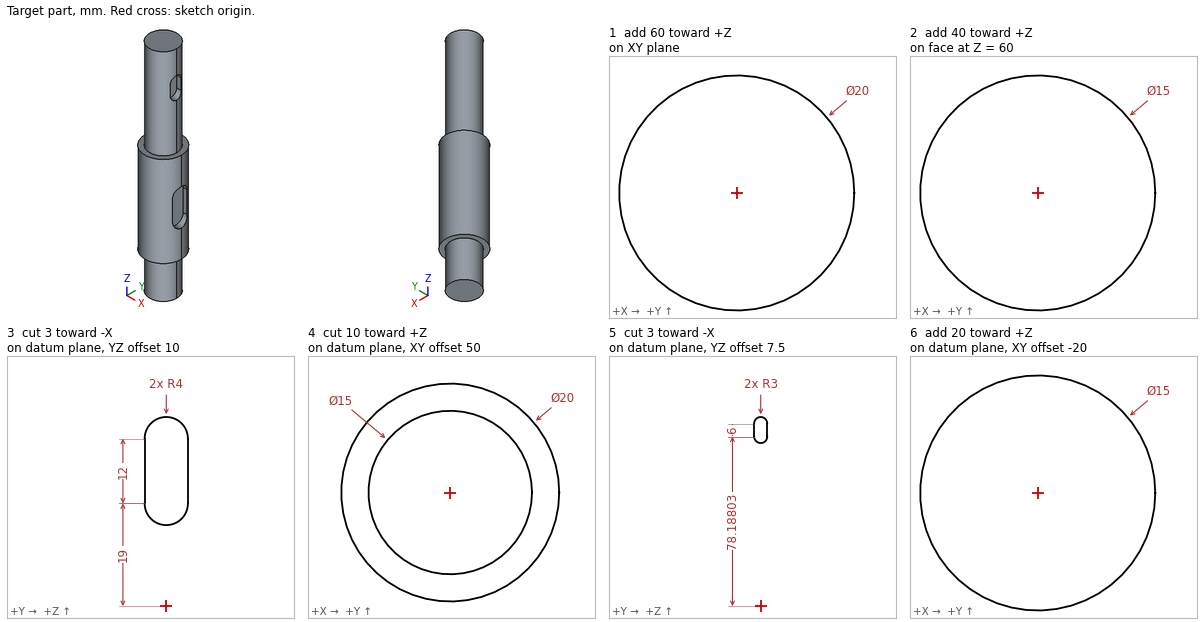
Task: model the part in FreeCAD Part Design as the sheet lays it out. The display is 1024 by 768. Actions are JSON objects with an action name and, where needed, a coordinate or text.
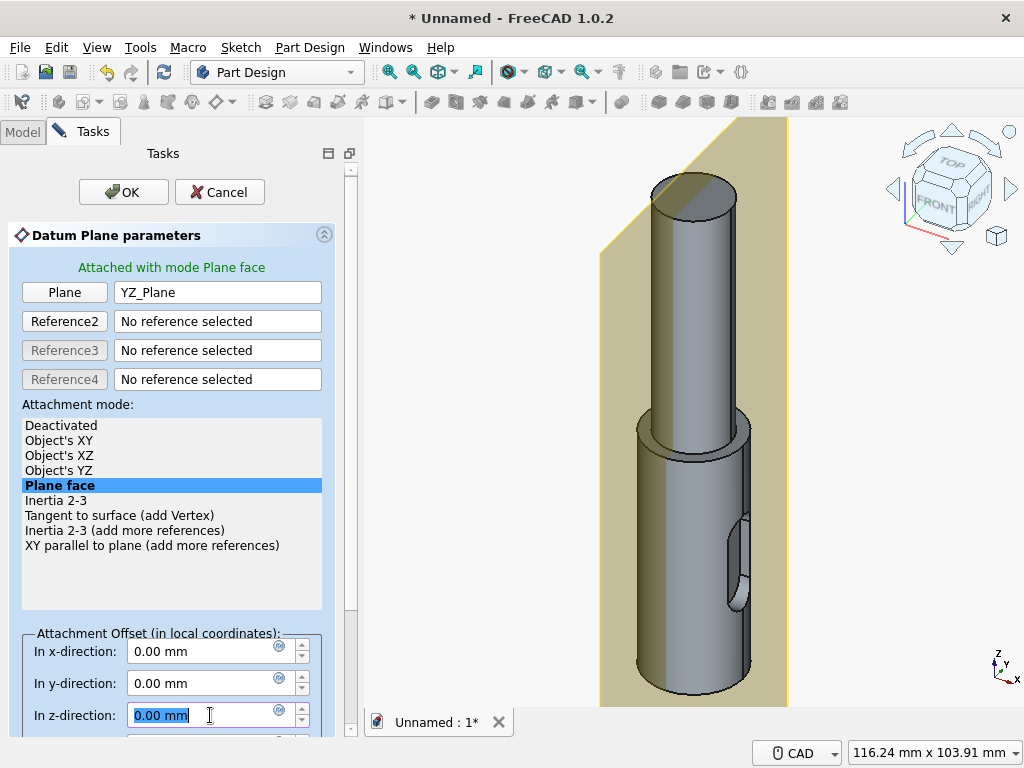
{"action": "type", "text": "7.5"}
{"action": "key", "text": "Tab"}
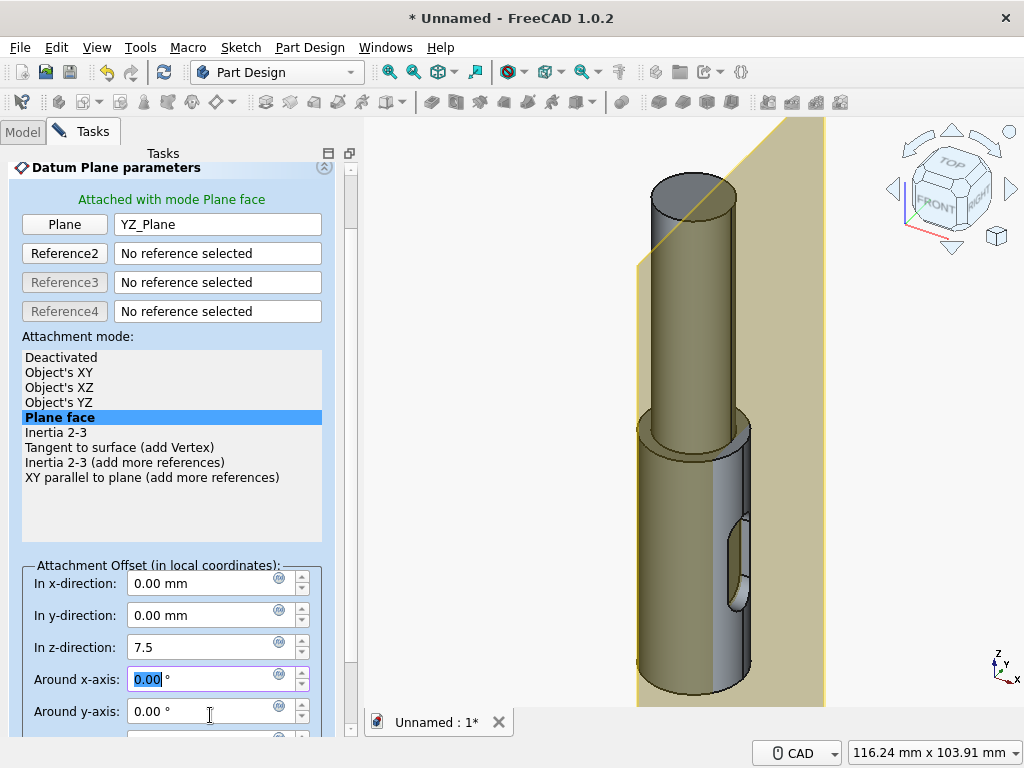
{"action": "scroll", "coordinate": [351, 450], "scroll_direction": "up", "scroll_amount": 2}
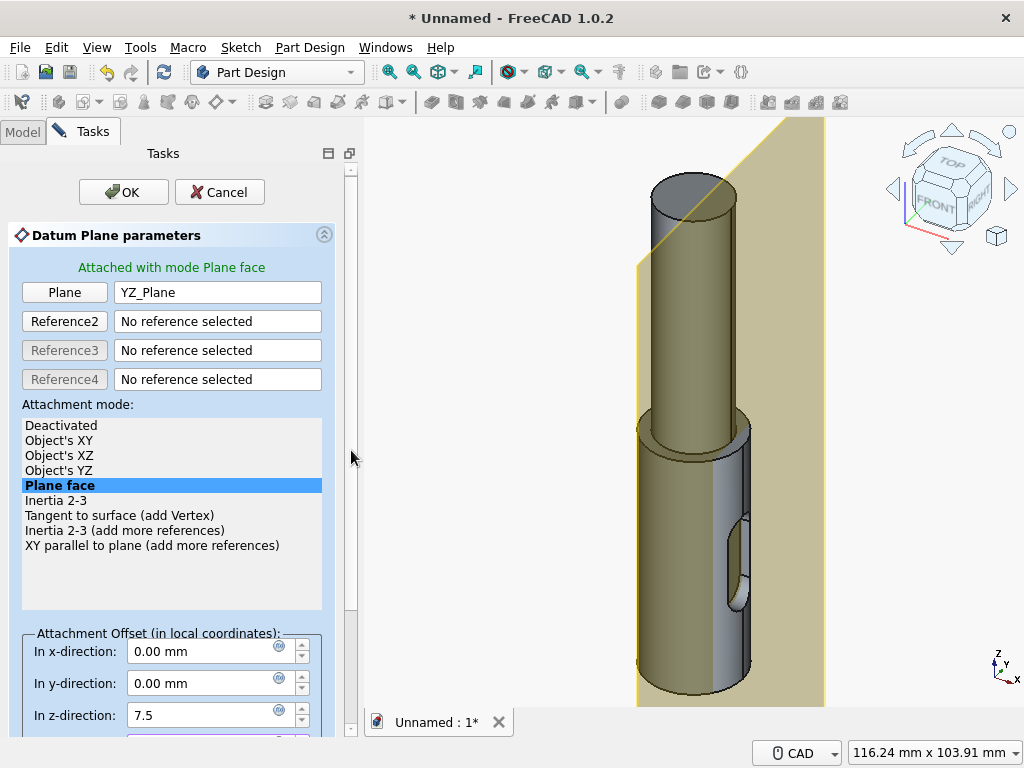
{"action": "left_click", "coordinate": [124, 192]}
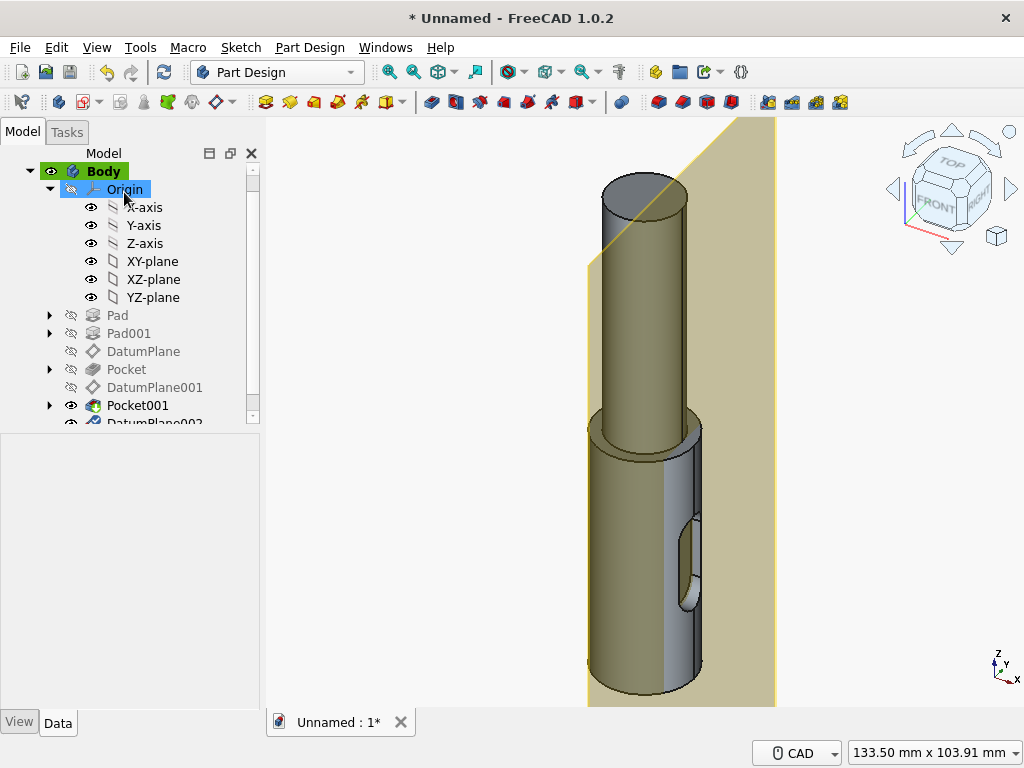
{"action": "left_click", "coordinate": [116, 423]}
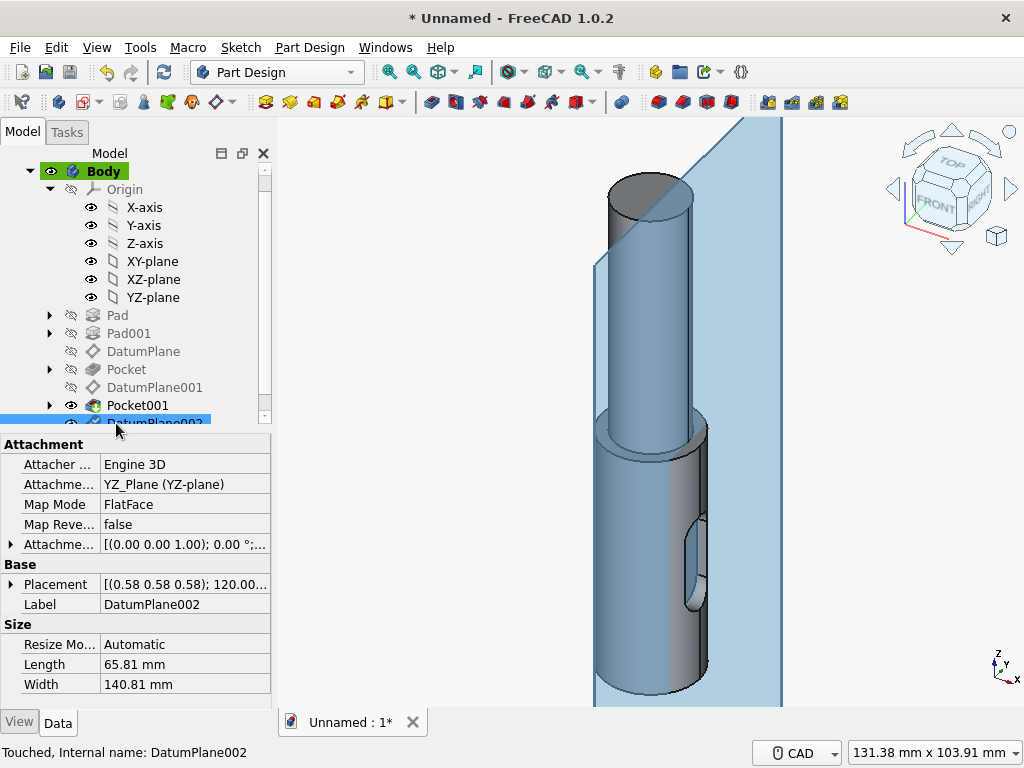
{"action": "left_click", "coordinate": [84, 102]}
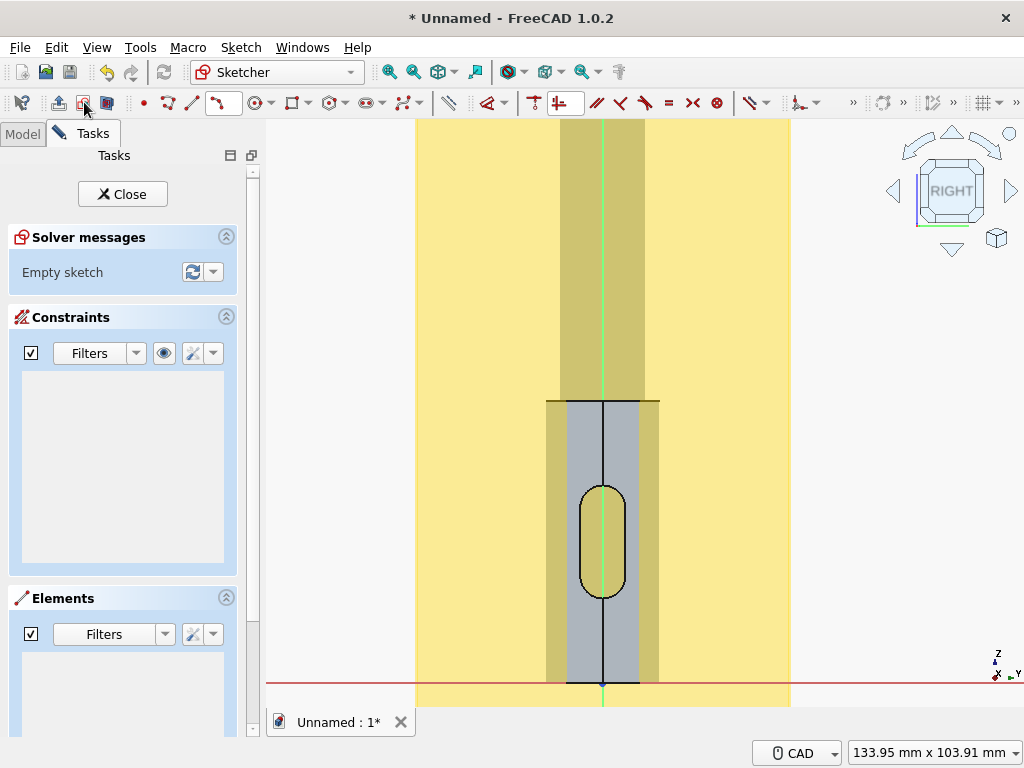
{"action": "left_click", "coordinate": [108, 104]}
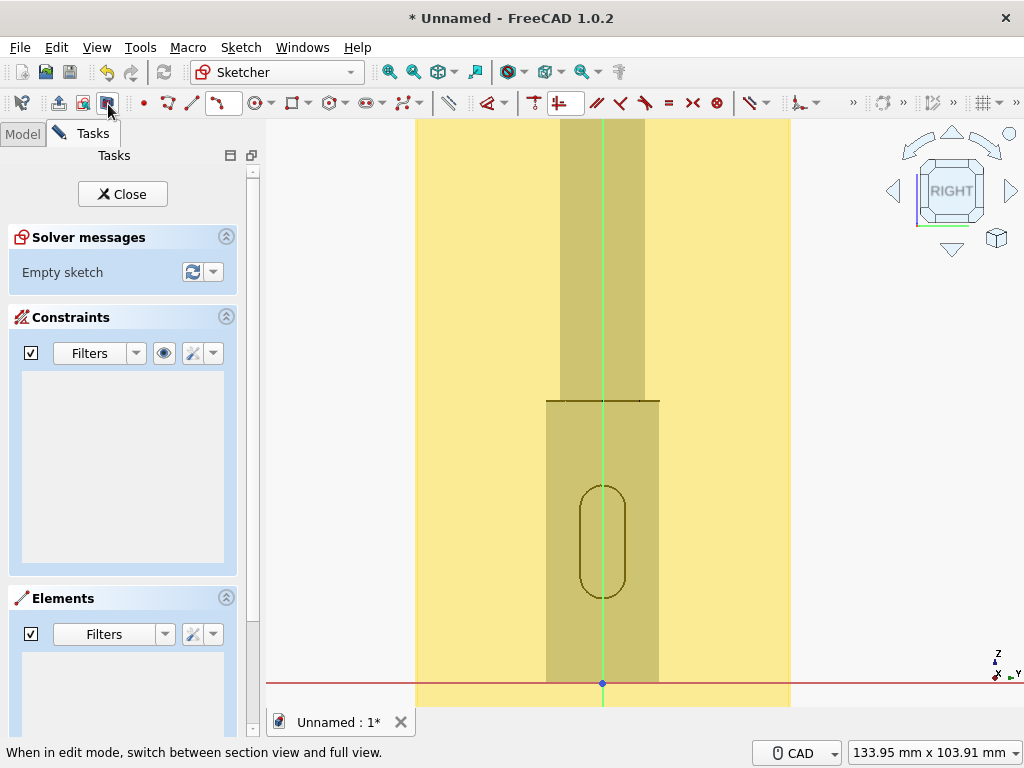
{"action": "scroll", "coordinate": [608, 187], "scroll_direction": "up", "scroll_amount": 9}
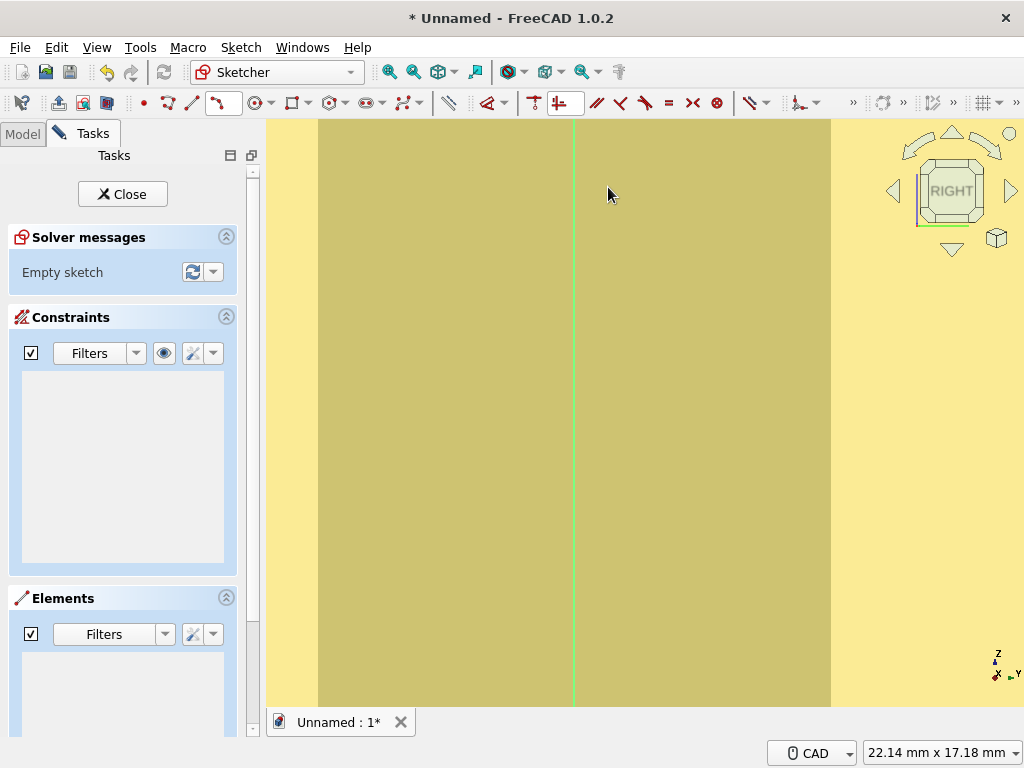
{"action": "left_click", "coordinate": [366, 104]}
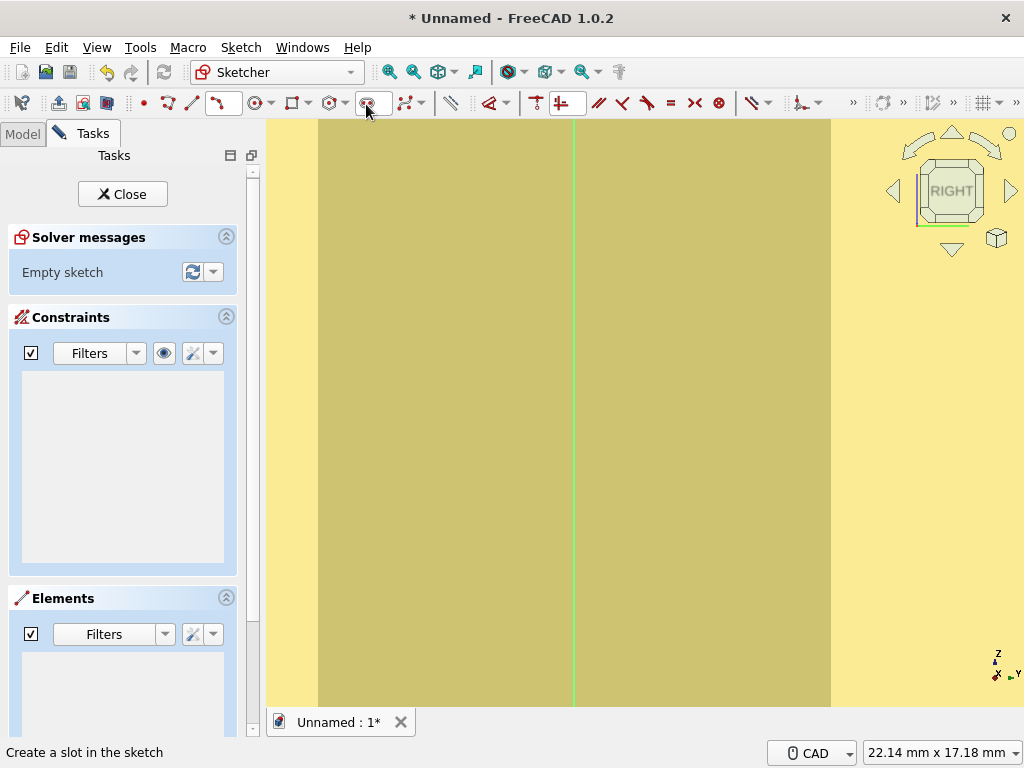
{"action": "left_click", "coordinate": [574, 513]}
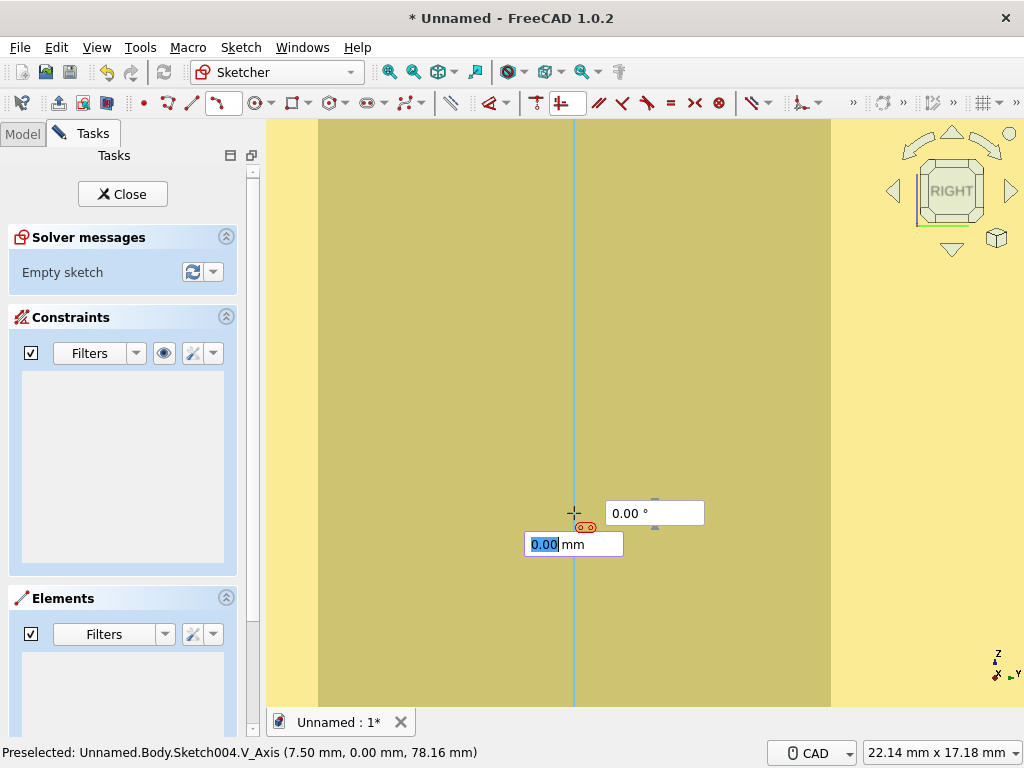
{"action": "left_click", "coordinate": [583, 308]}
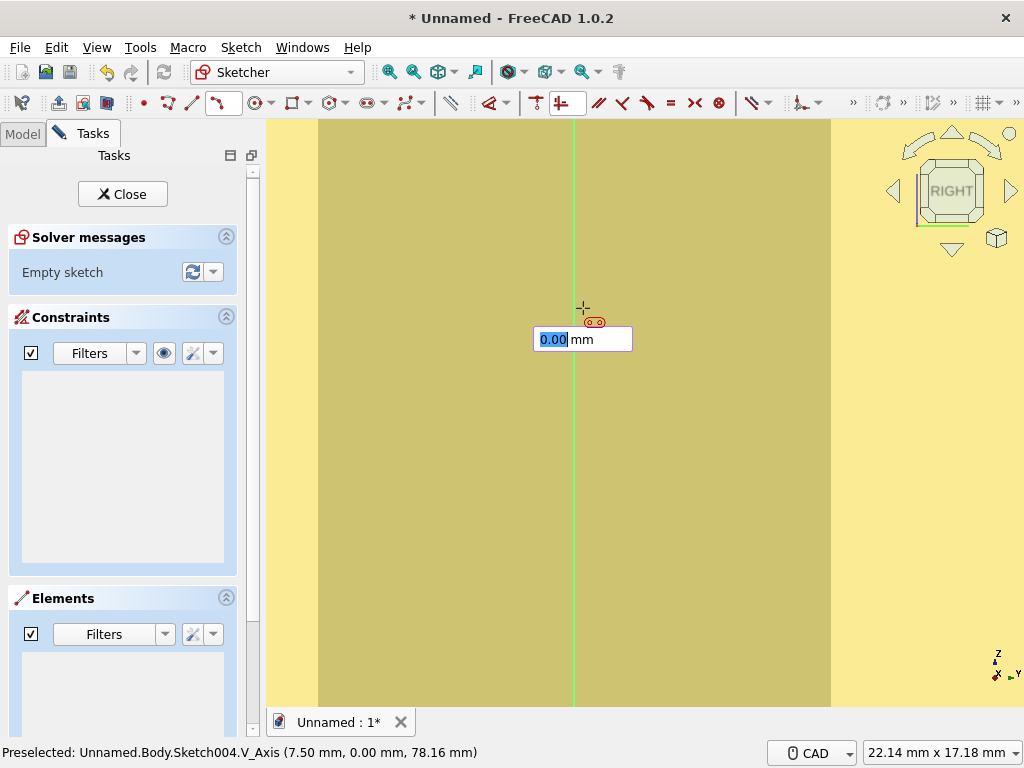
{"action": "left_click", "coordinate": [677, 410]}
{"action": "key", "text": "Escape"}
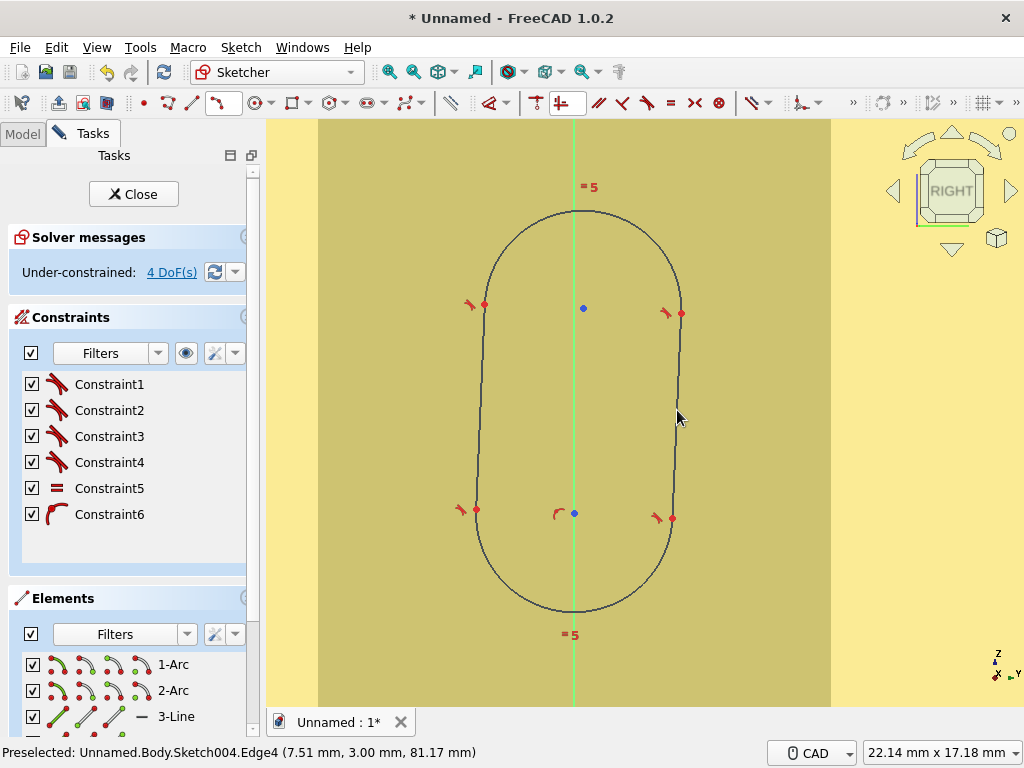
{"action": "left_click", "coordinate": [479, 448]}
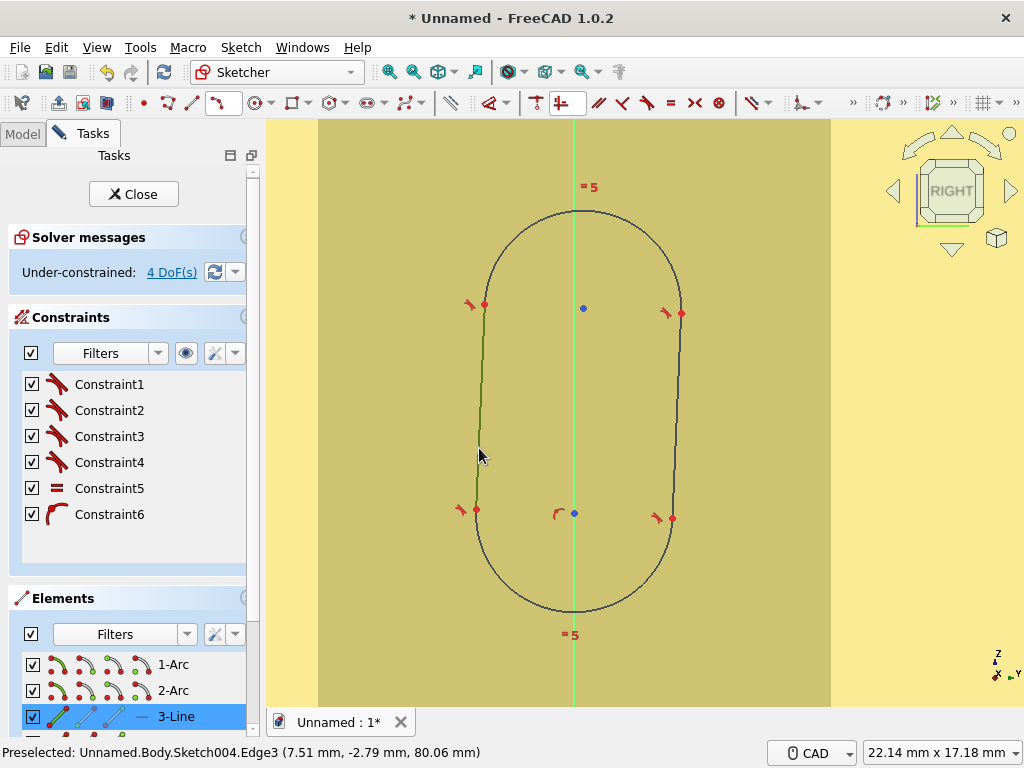
{"action": "left_click", "coordinate": [580, 104]}